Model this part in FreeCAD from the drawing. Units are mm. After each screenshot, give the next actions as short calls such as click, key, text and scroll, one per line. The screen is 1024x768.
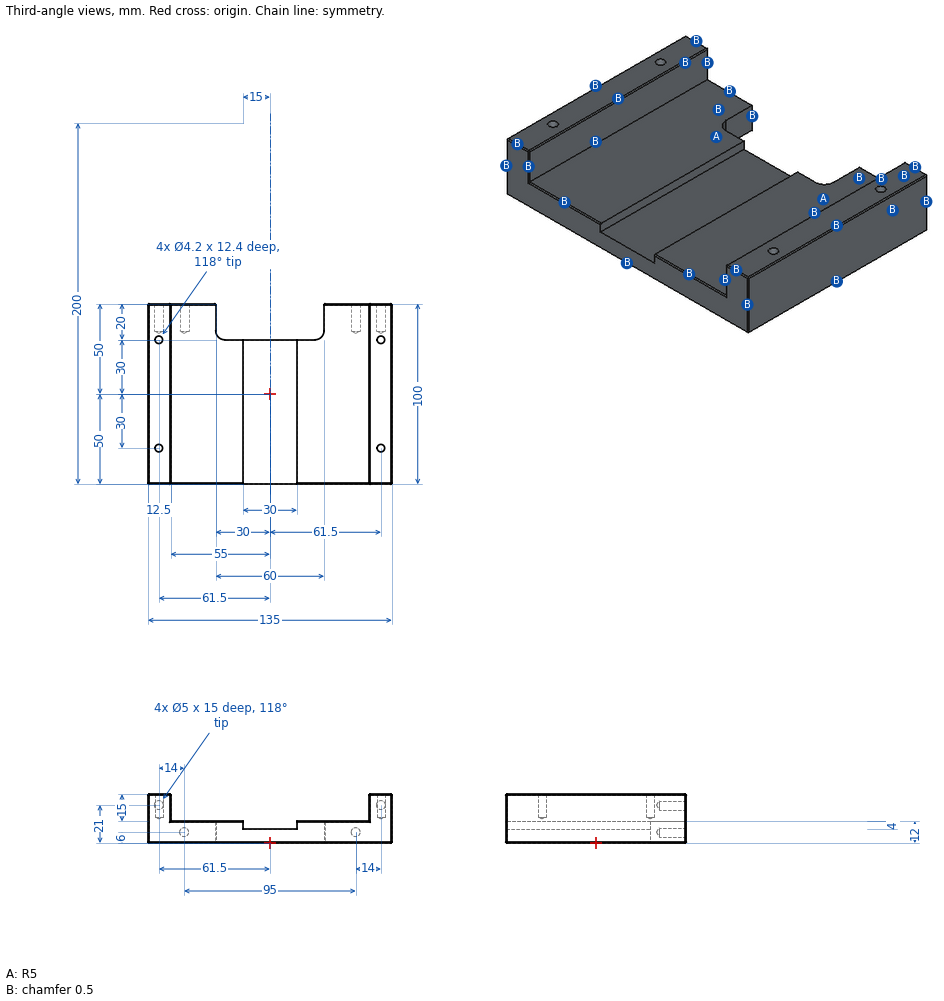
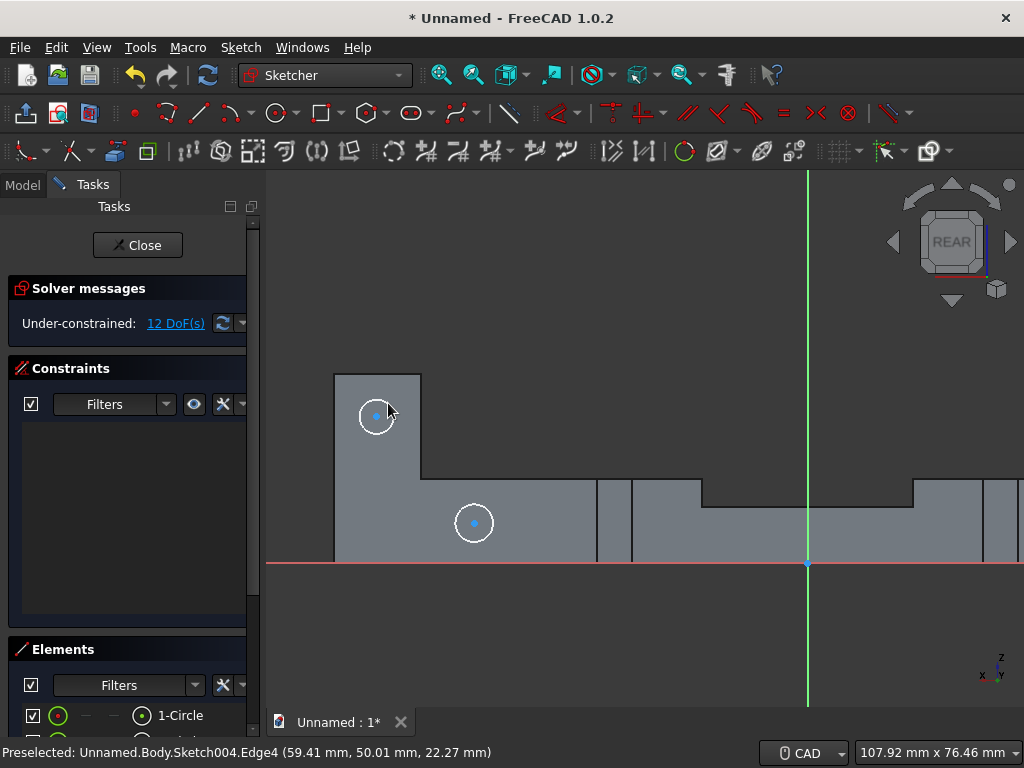
scroll(388, 404, down, 4)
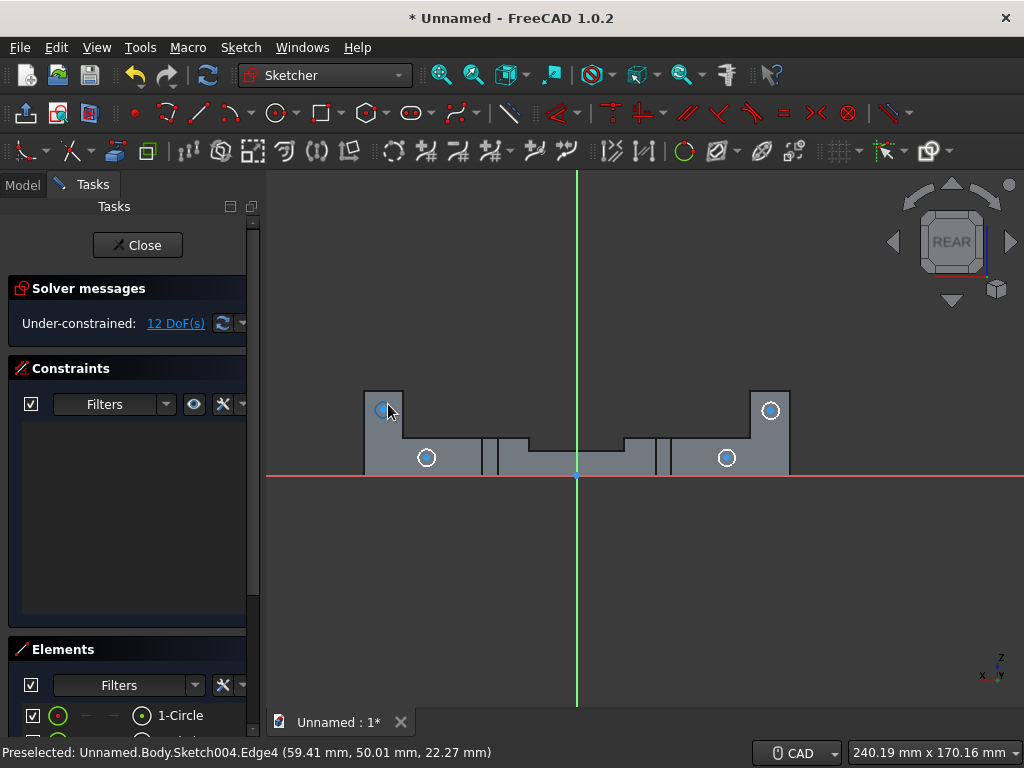
scroll(777, 405, up, 3)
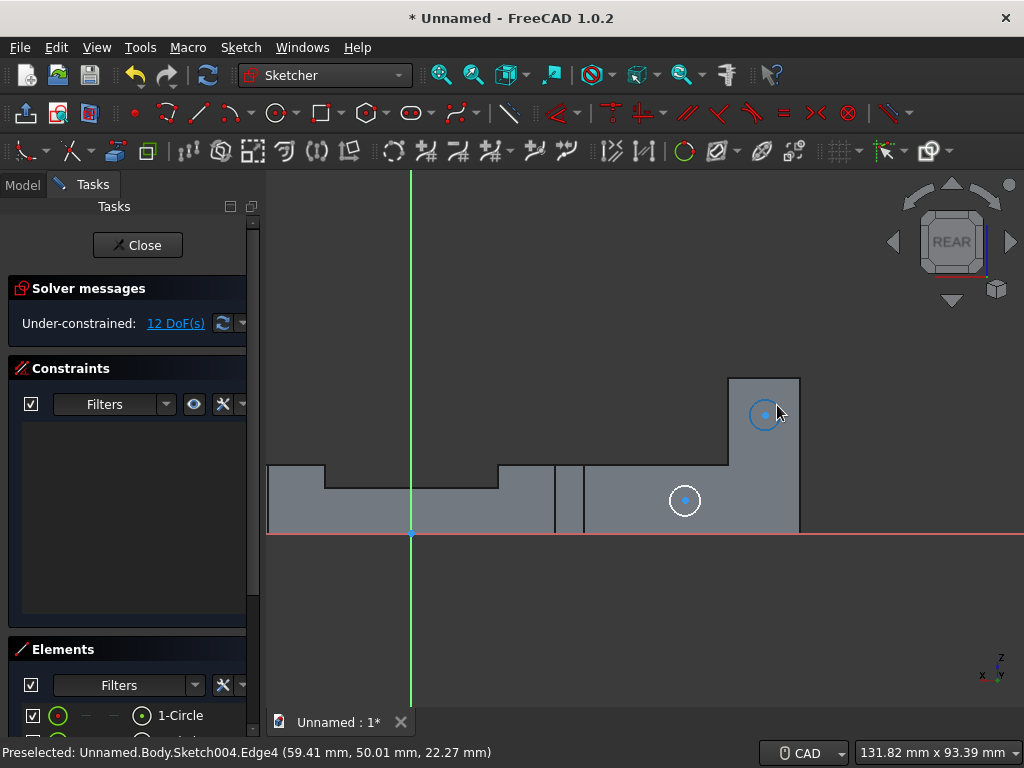
click(776, 404)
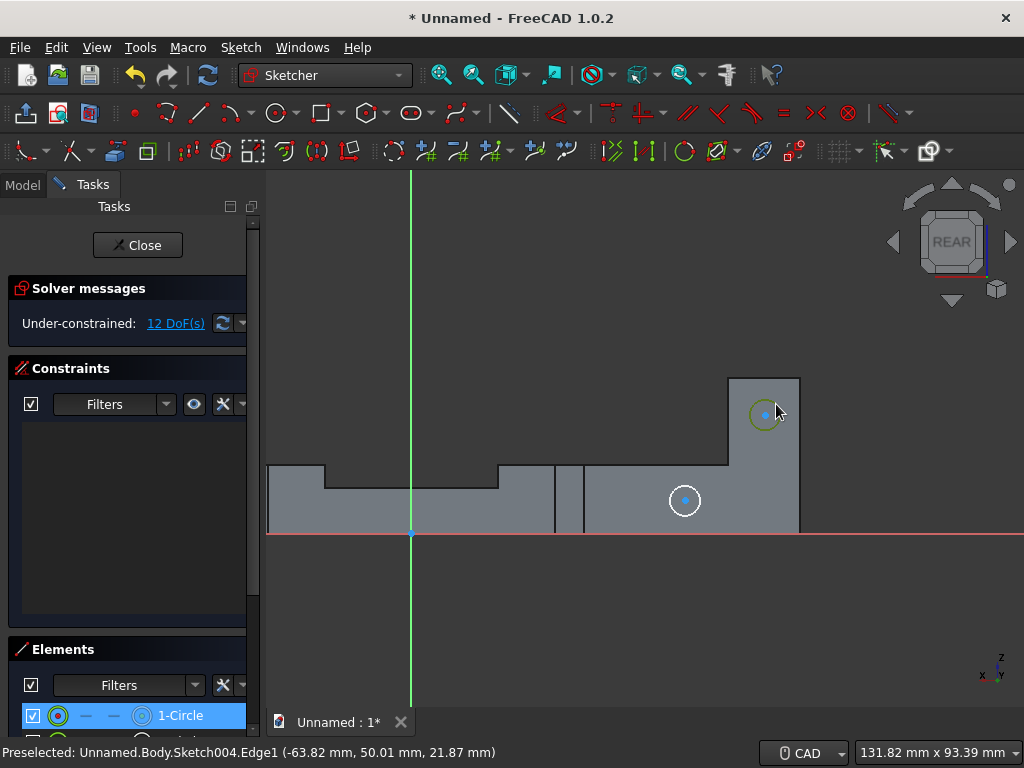
click(696, 490)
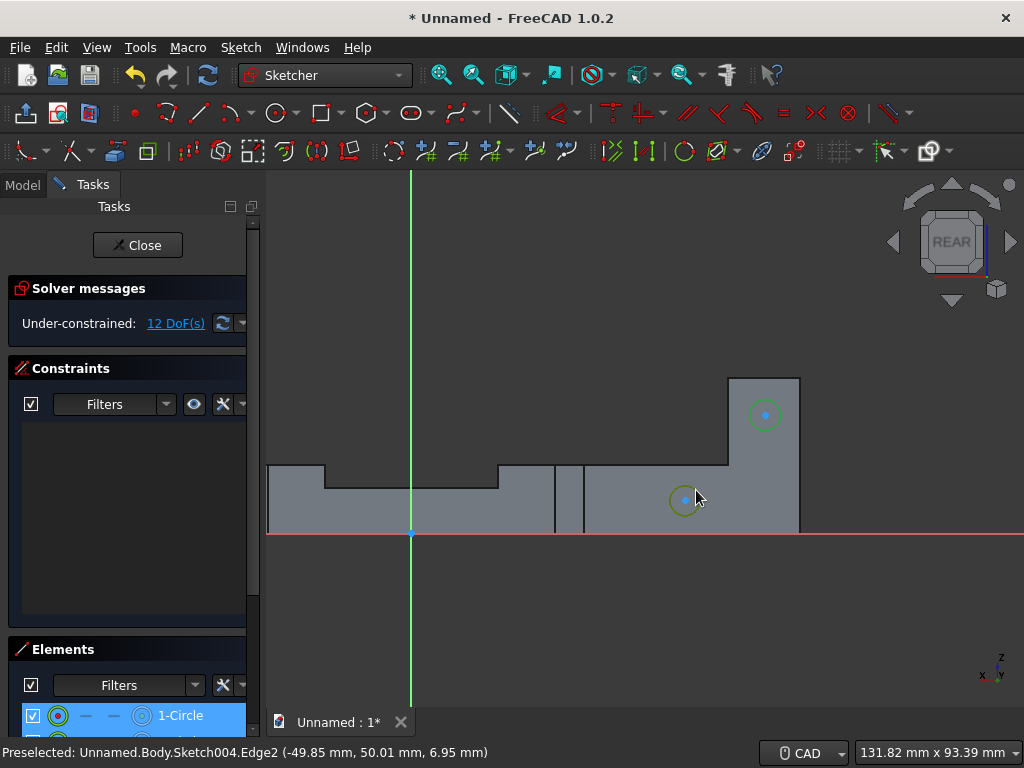
scroll(777, 405, down, 3)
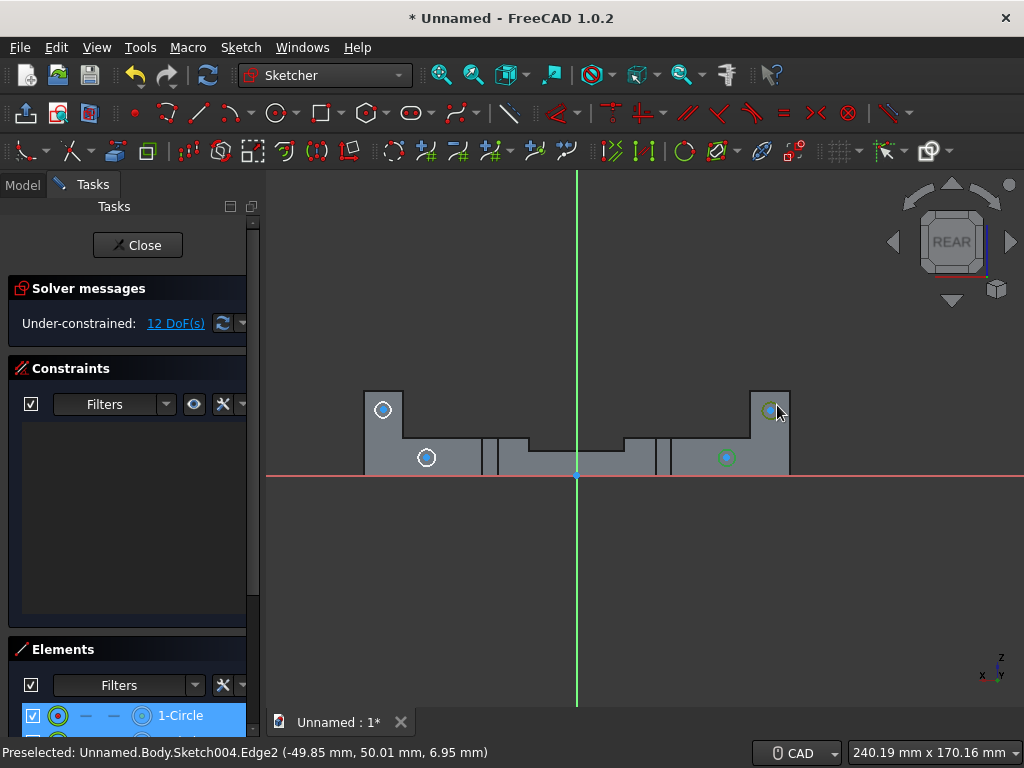
scroll(433, 452, up, 3)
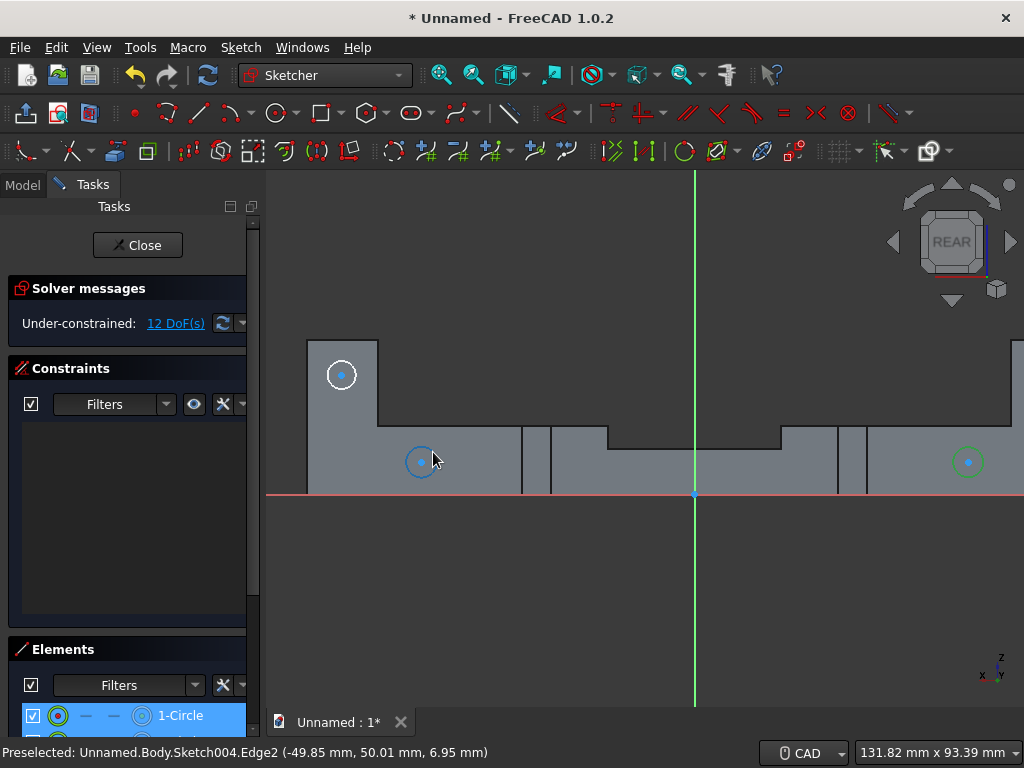
click(432, 451)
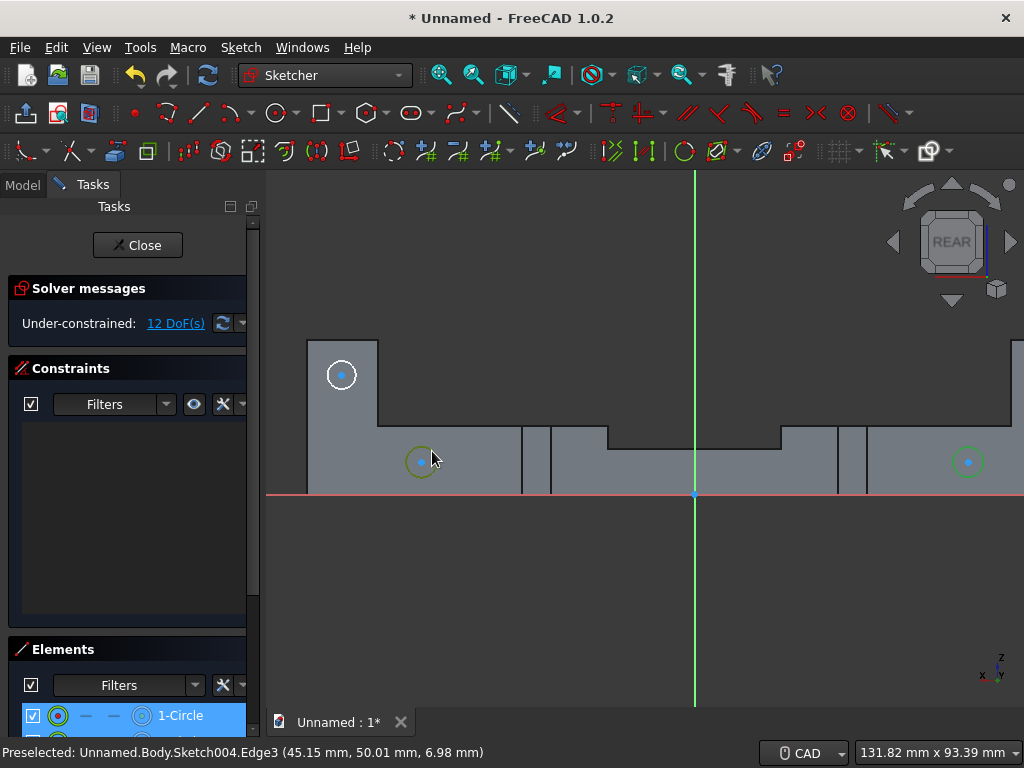
click(352, 365)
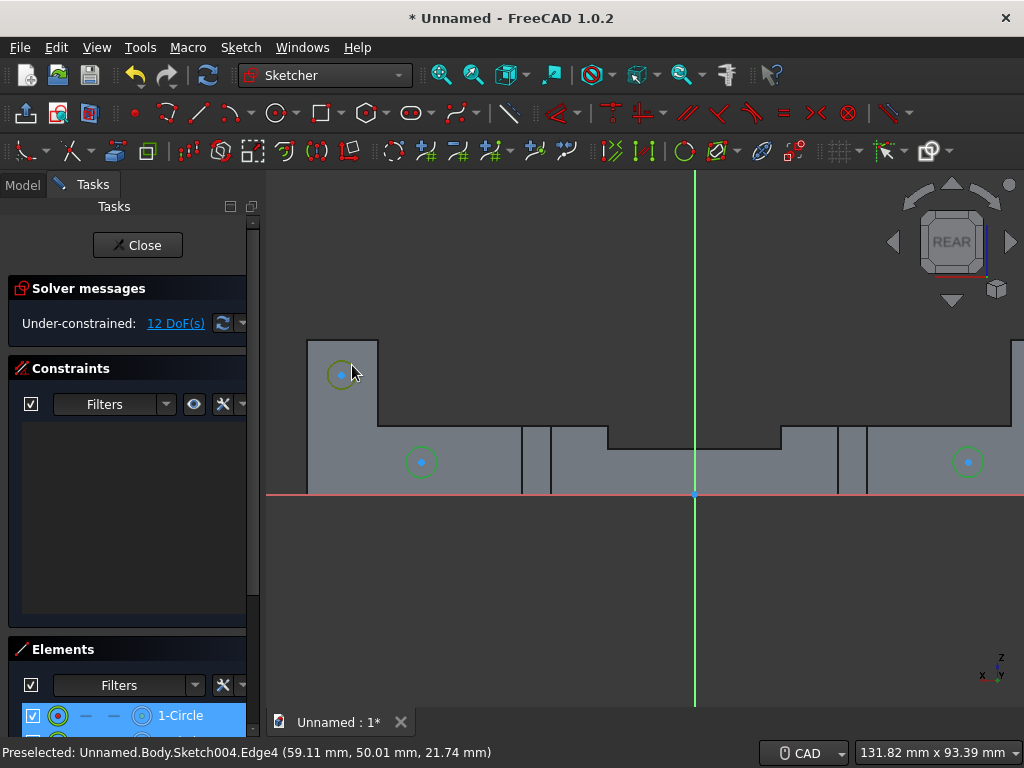
key(e)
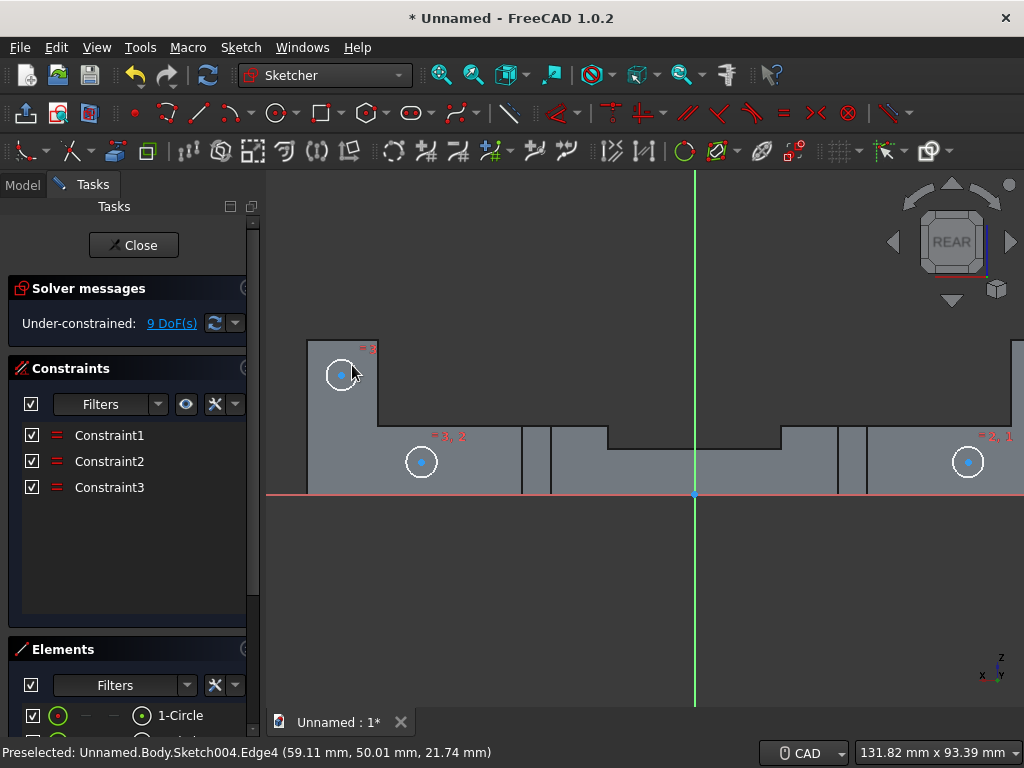
scroll(433, 452, down, 3)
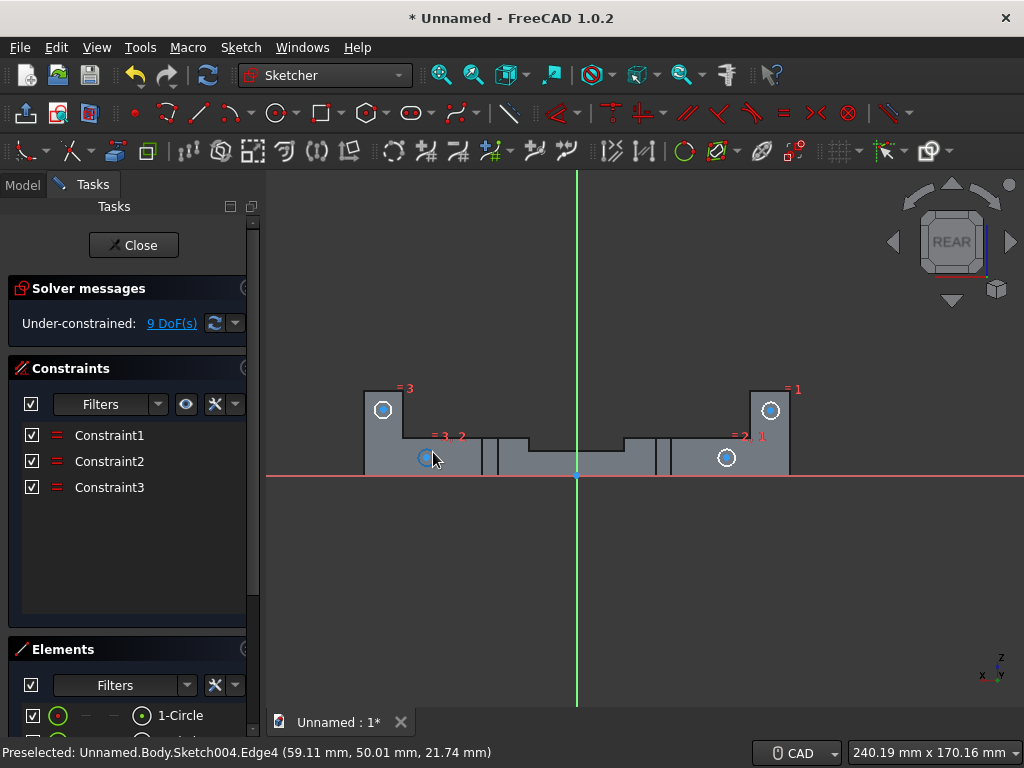
click(727, 458)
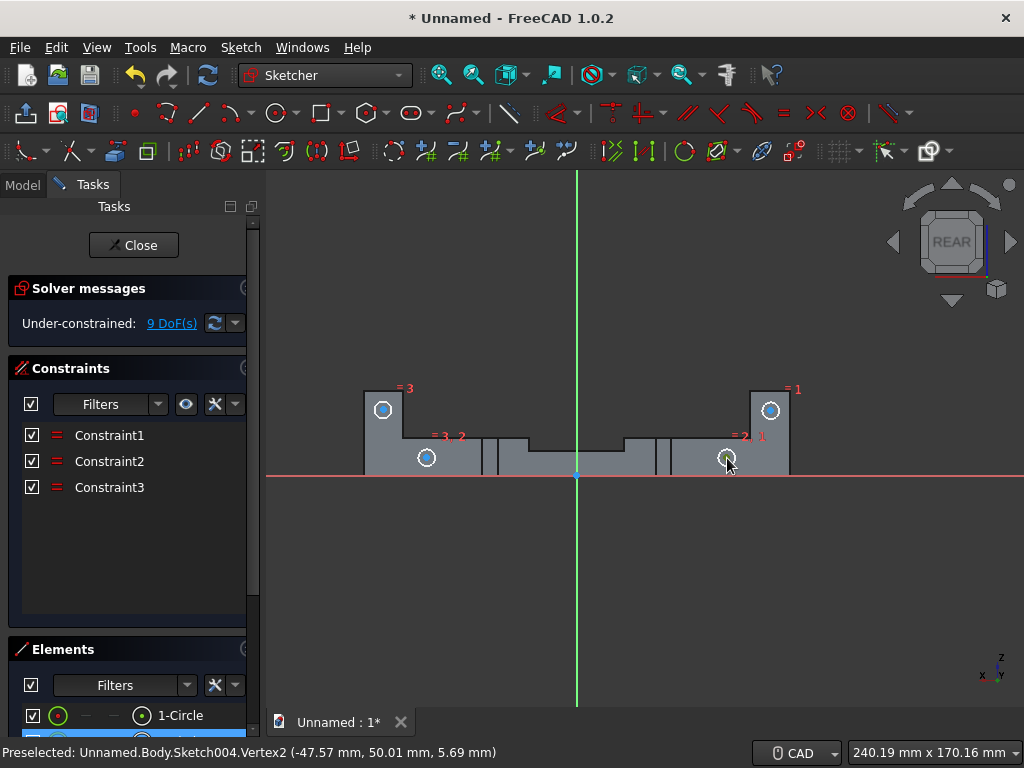
click(427, 458)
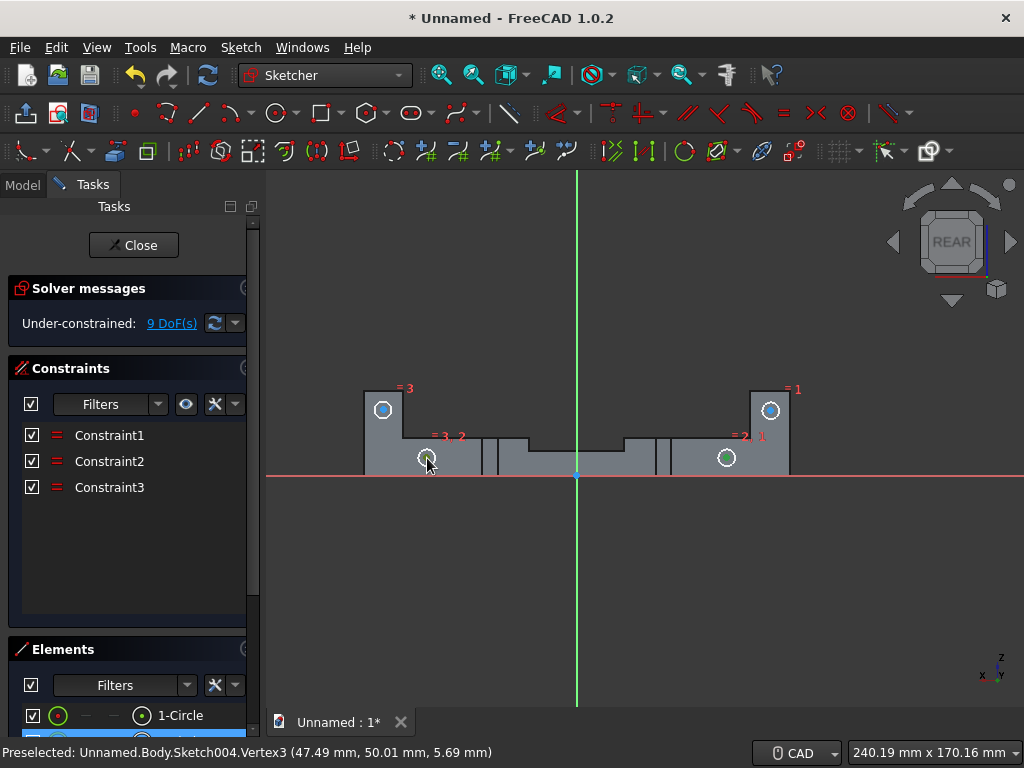
click(666, 114)